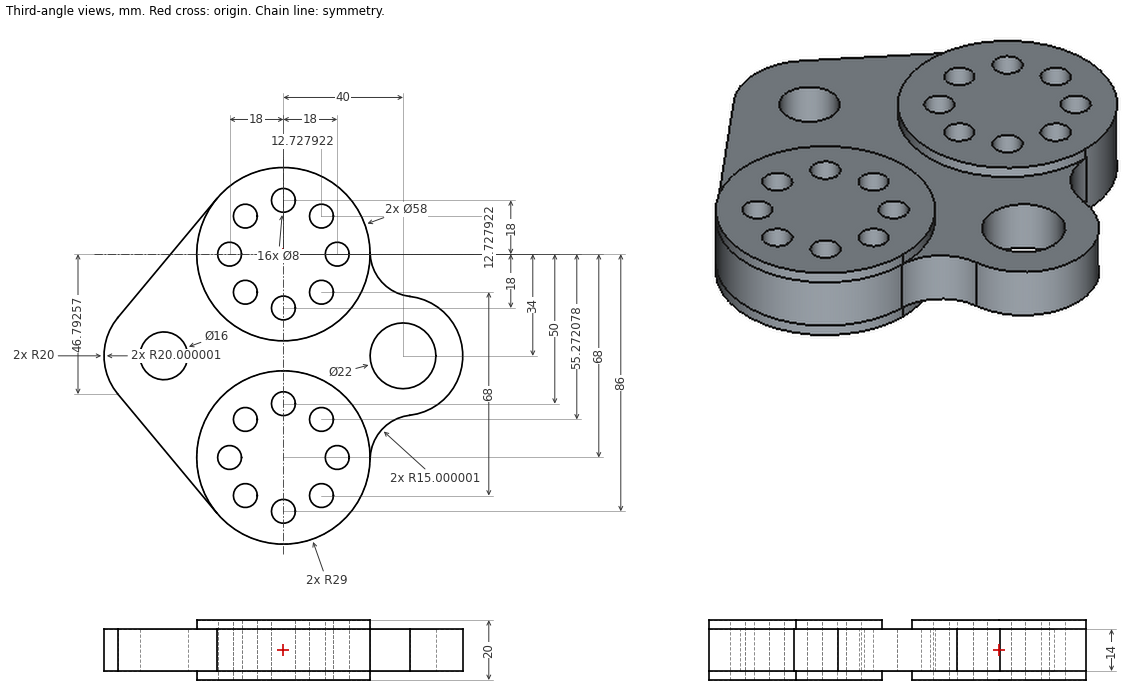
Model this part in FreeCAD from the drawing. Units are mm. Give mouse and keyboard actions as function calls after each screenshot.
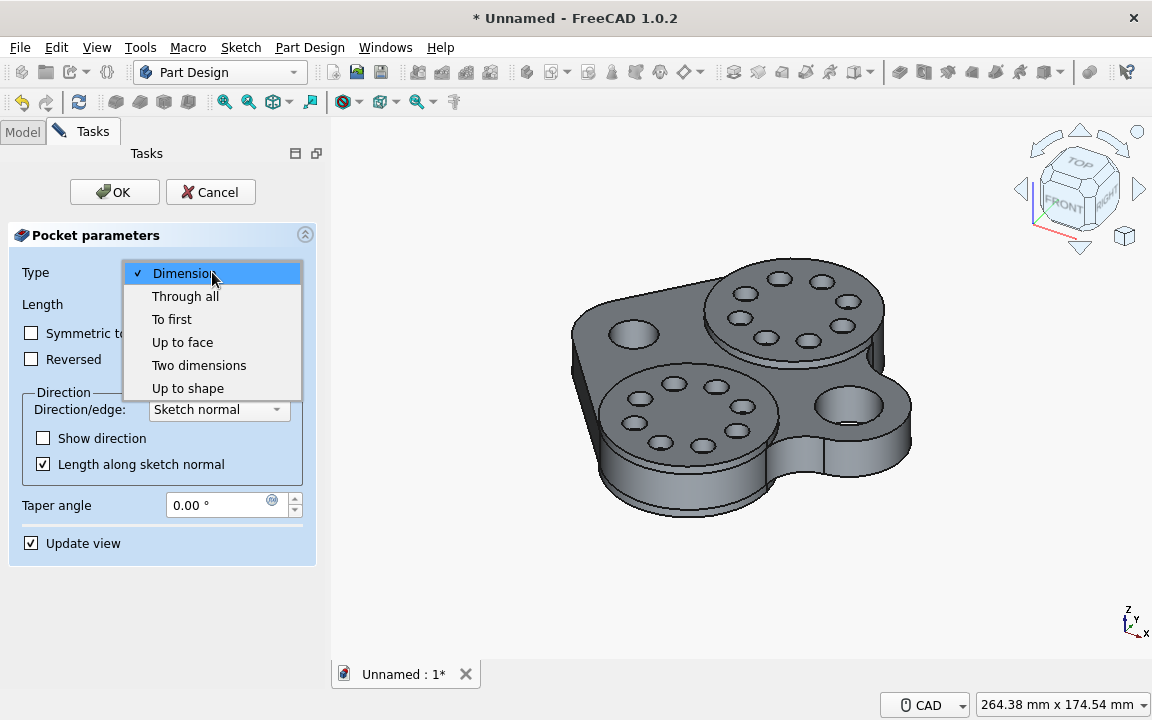
click(212, 296)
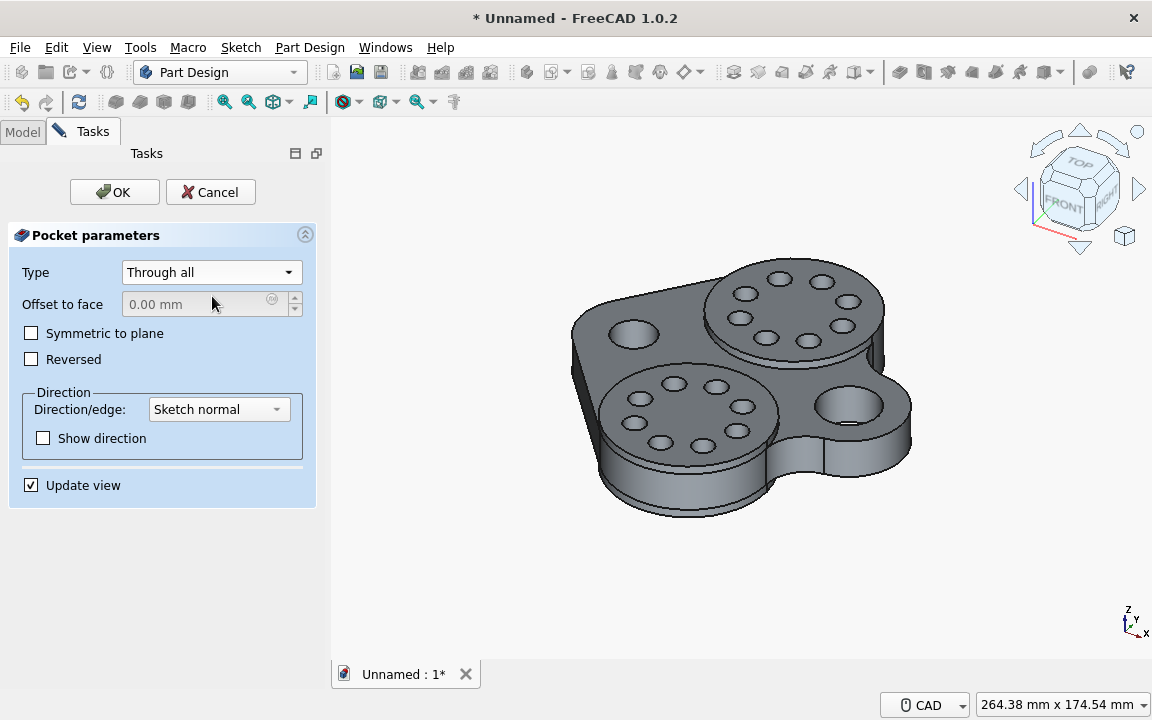
click(115, 192)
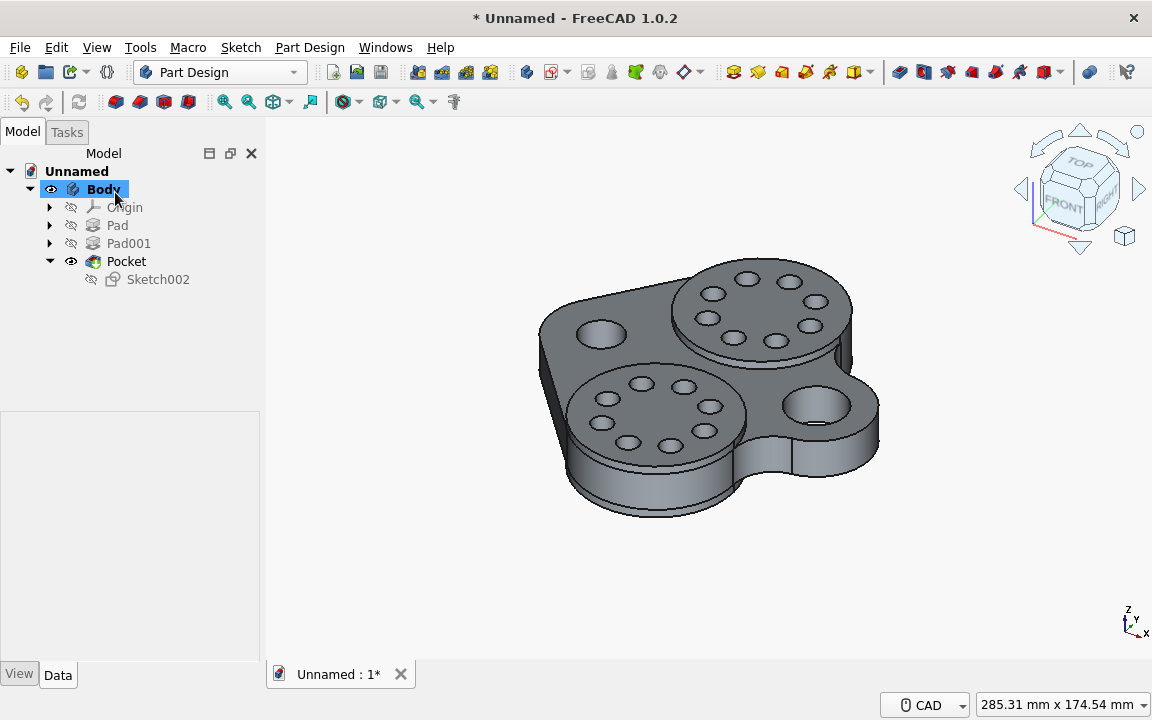
key(0)